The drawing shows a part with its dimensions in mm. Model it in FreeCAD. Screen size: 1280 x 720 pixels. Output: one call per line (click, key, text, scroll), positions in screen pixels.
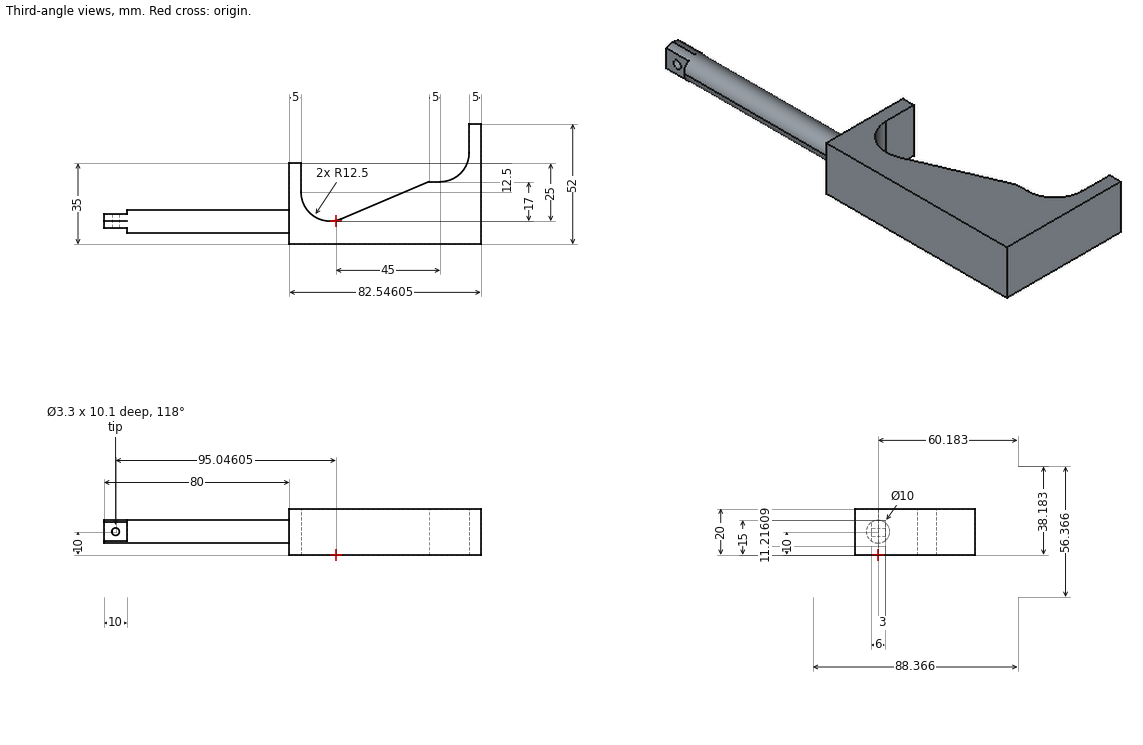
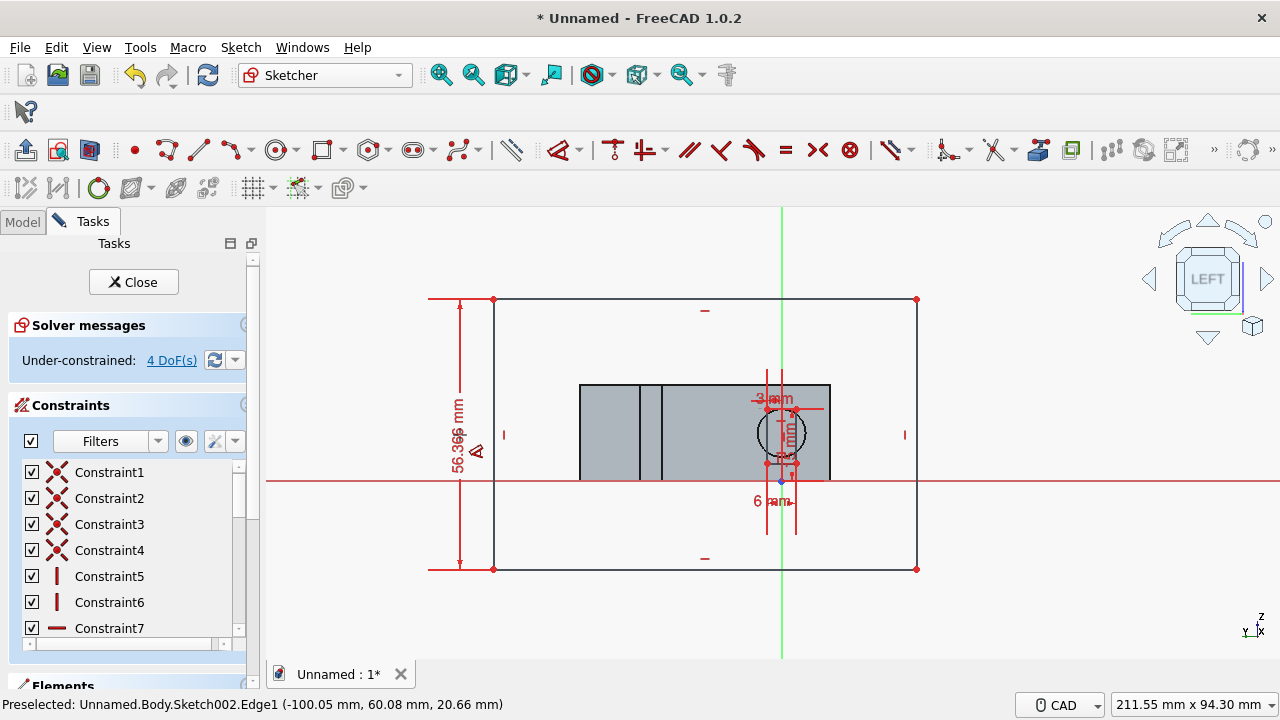
click(621, 570)
click(705, 604)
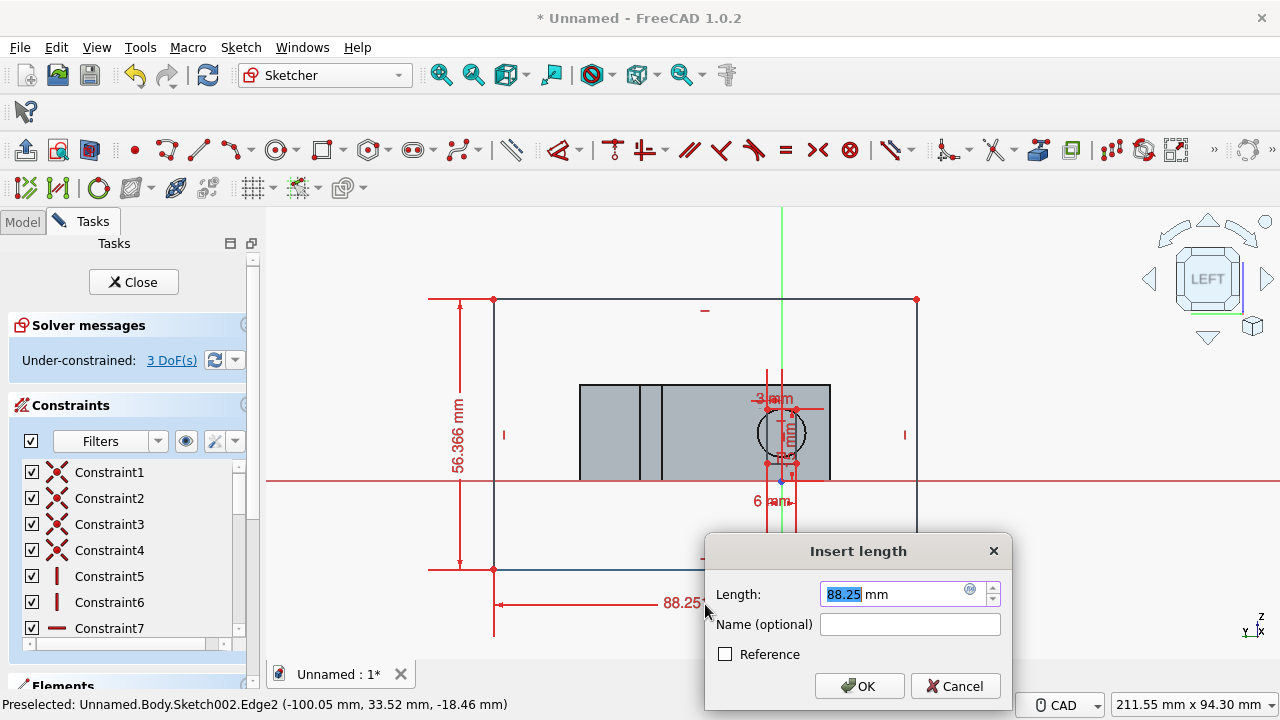
text(88.366)
key(Return)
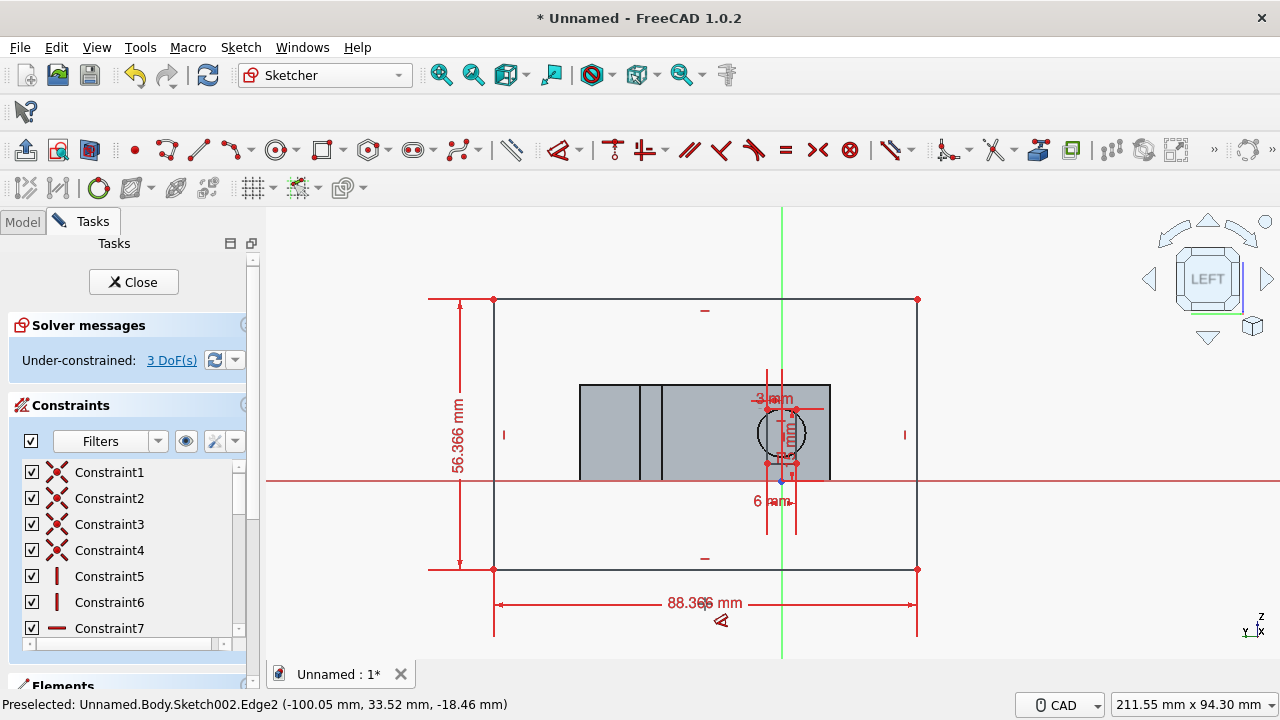
click(494, 299)
click(638, 265)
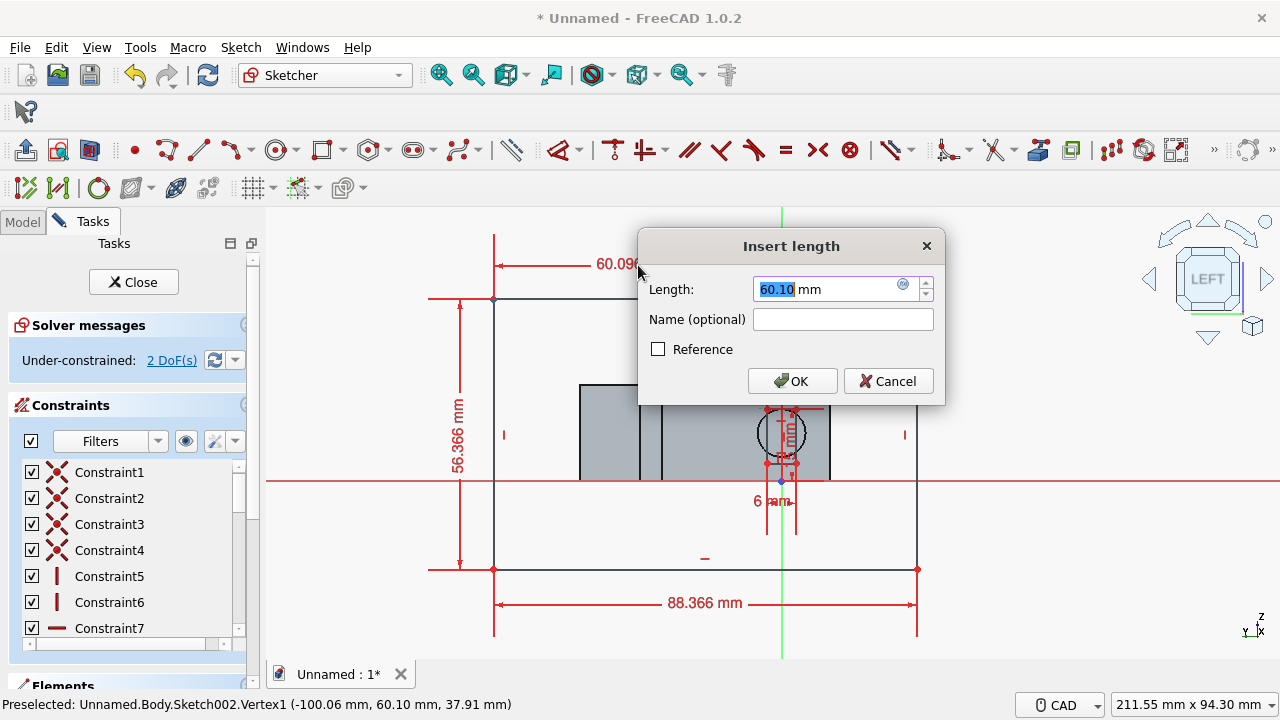
text(60.183)
key(Return)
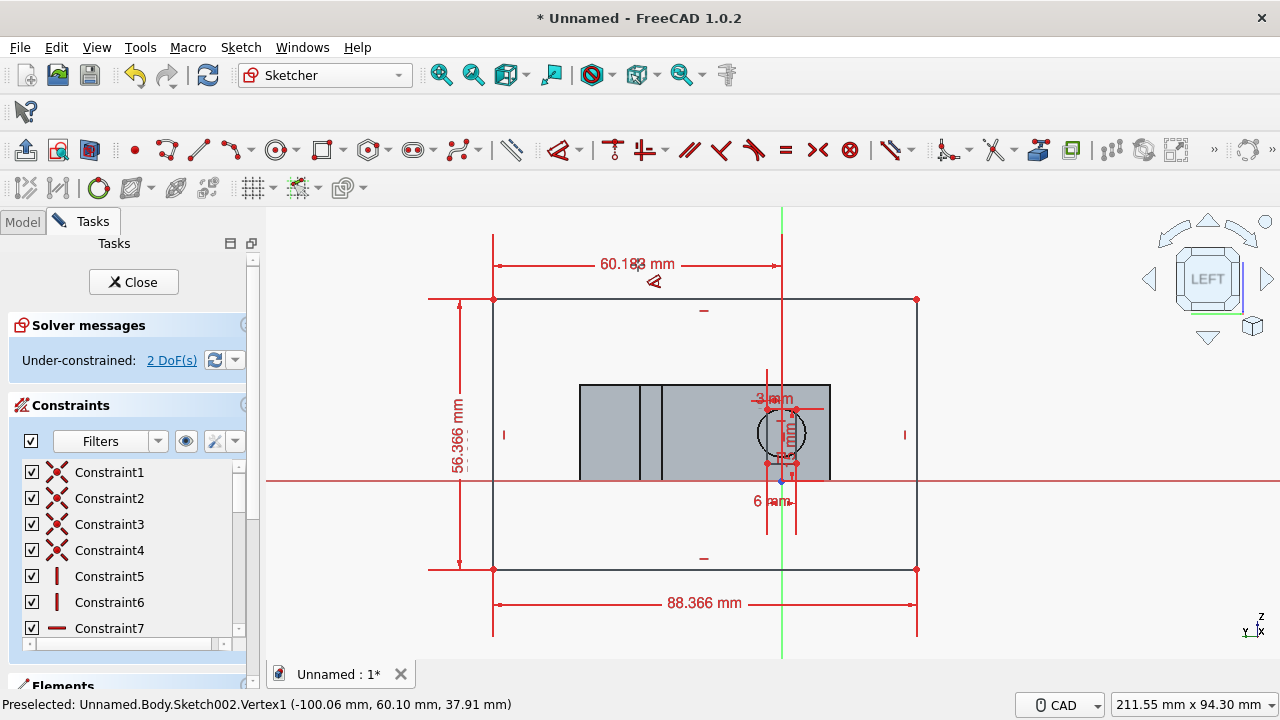
click(493, 299)
click(459, 390)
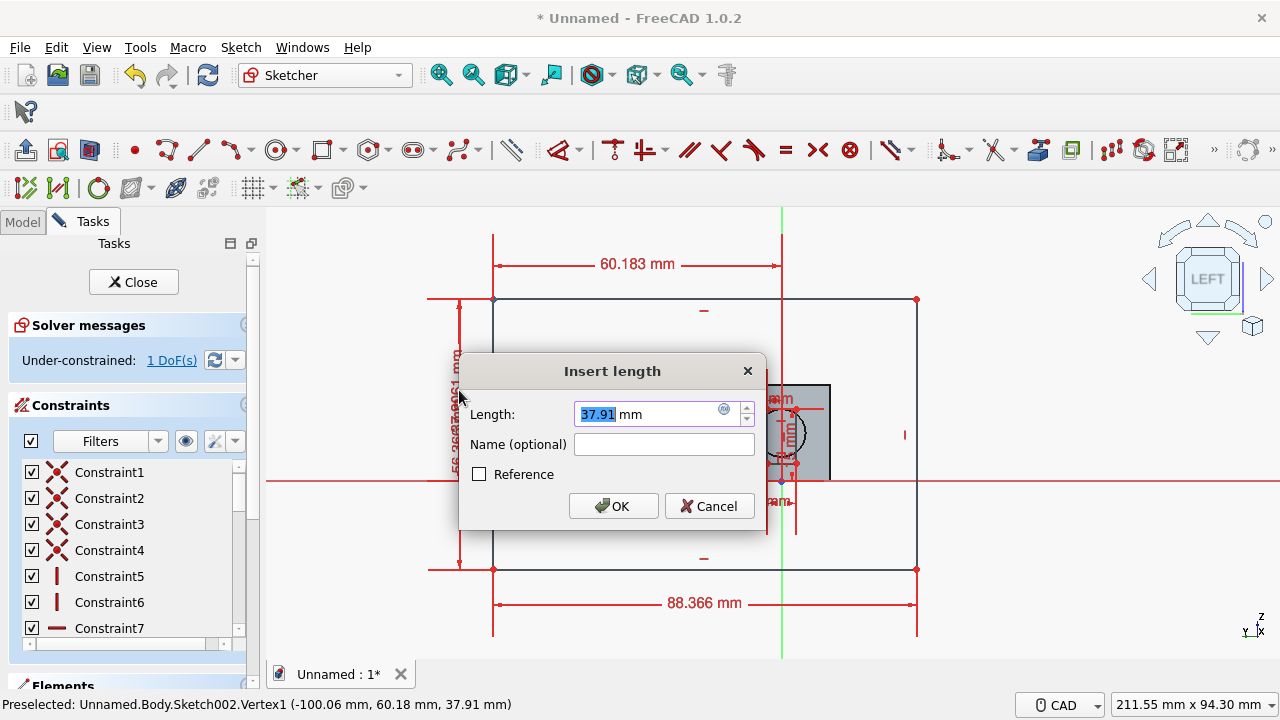
text(38.183)
key(Return)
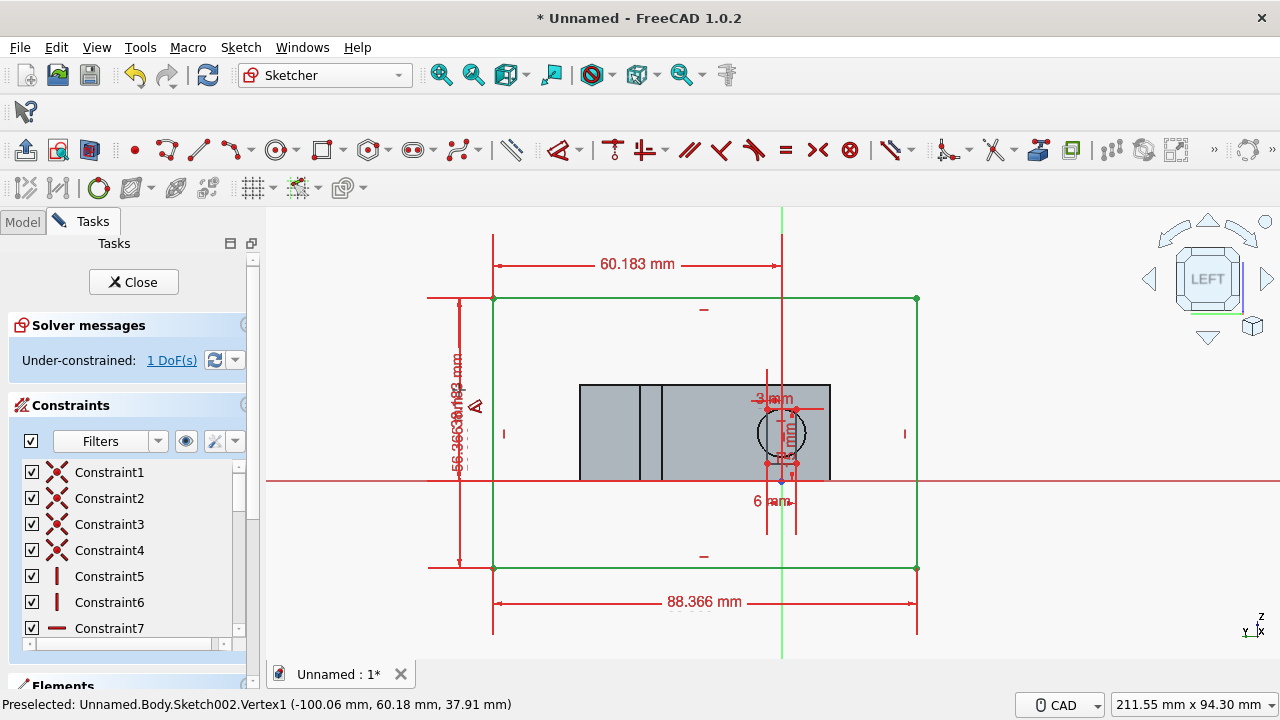
click(767, 425)
click(733, 424)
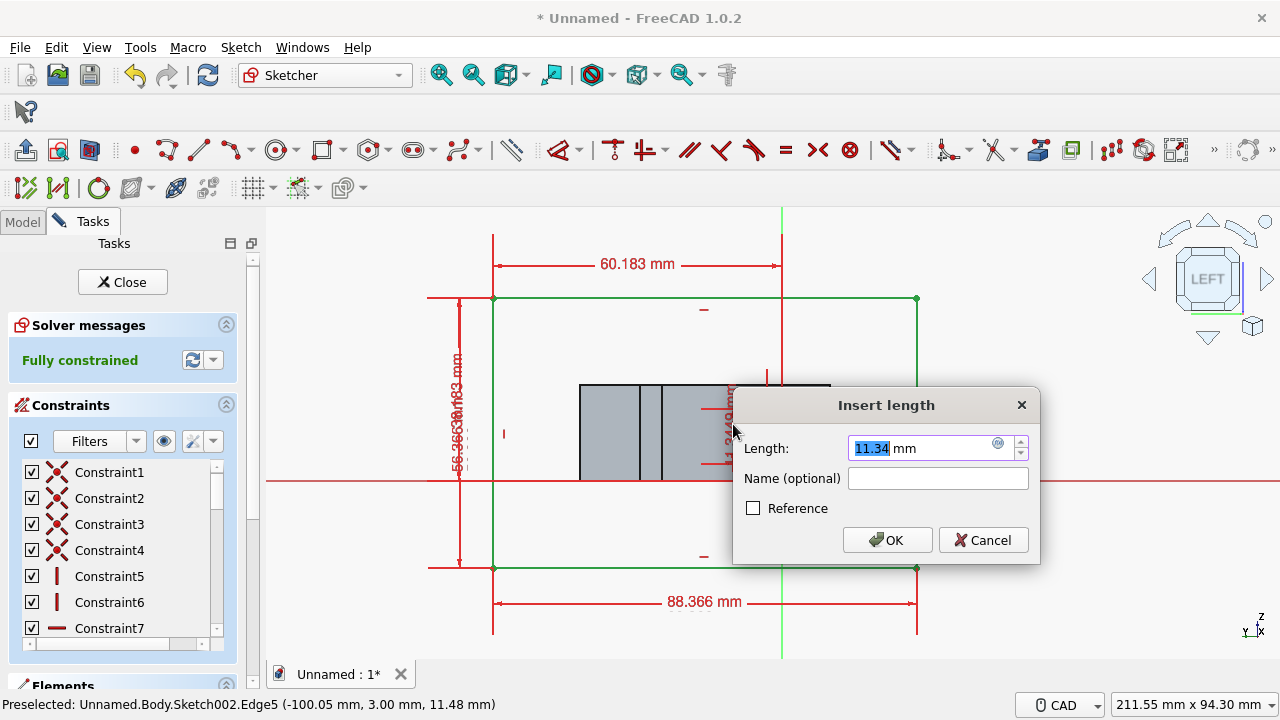
text(11.21609)
key(Return)
key(Escape)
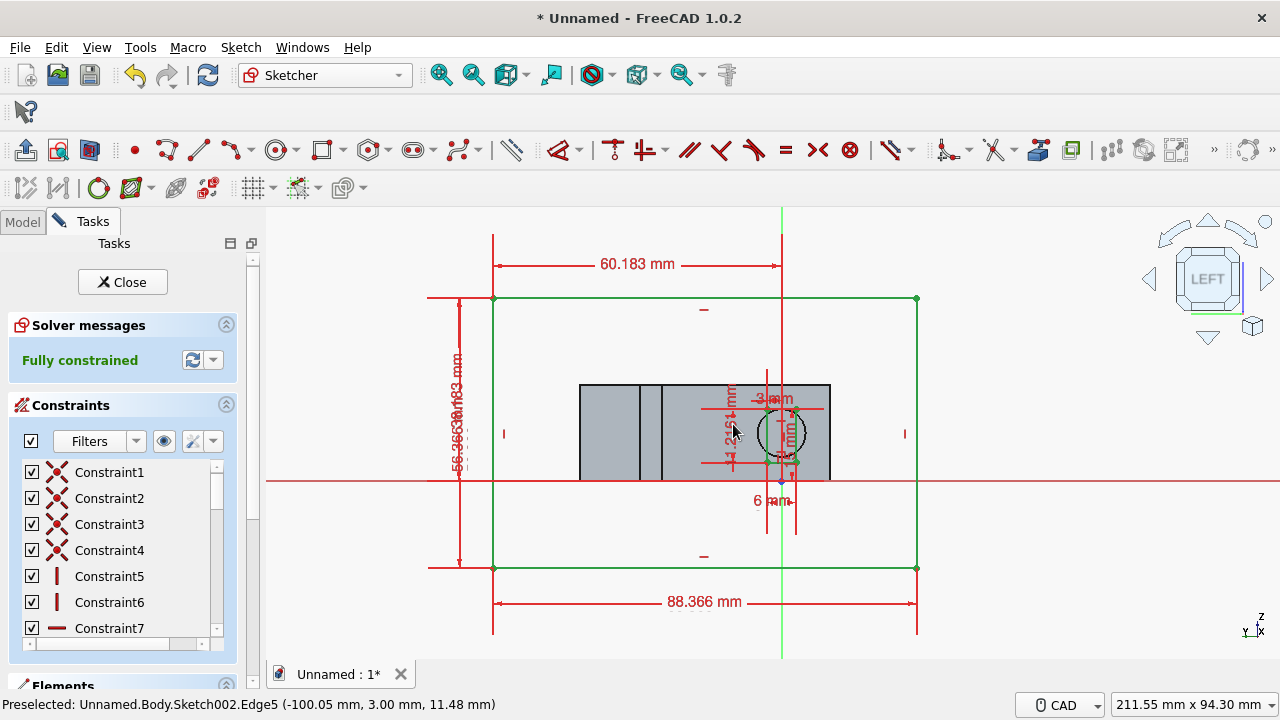
click(123, 282)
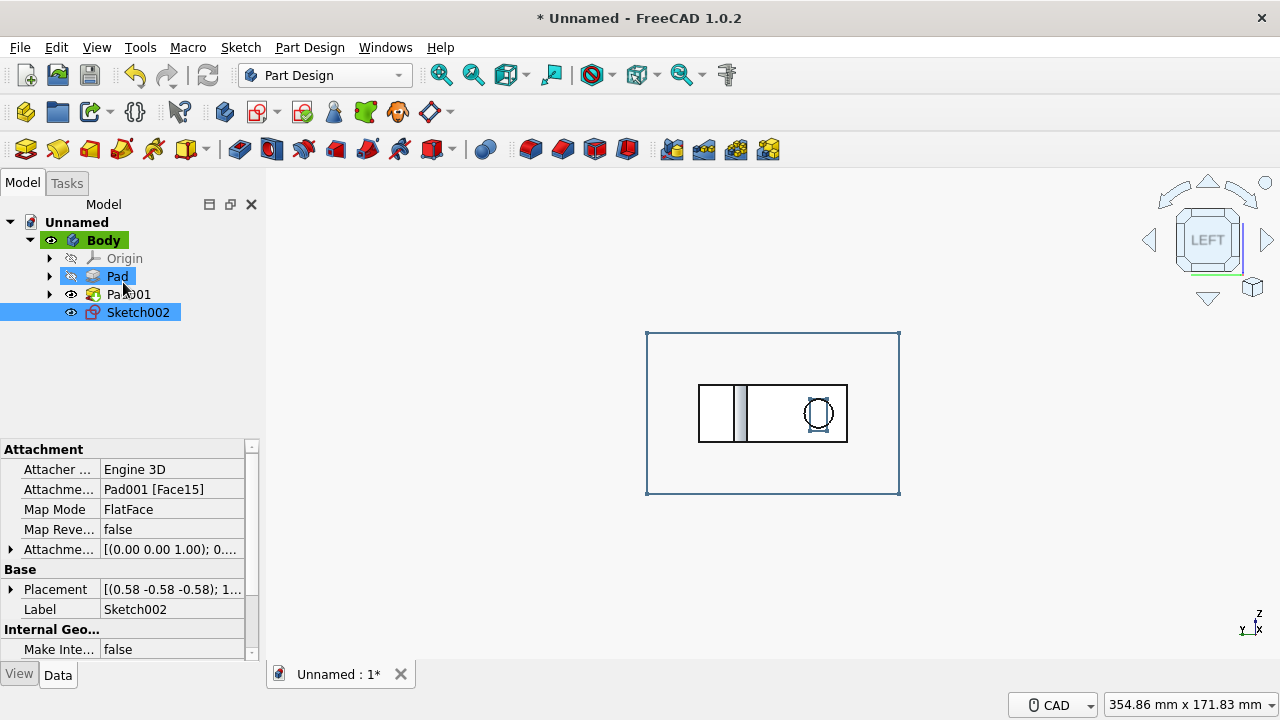
click(240, 150)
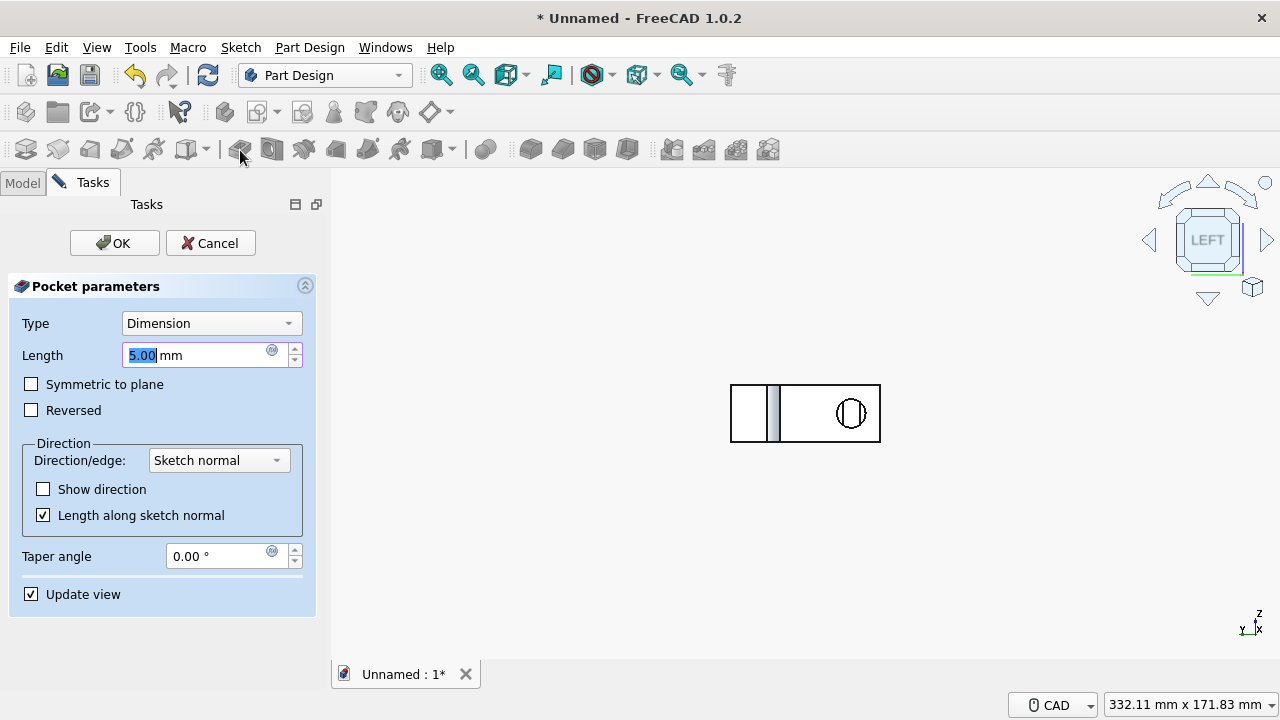
text(10)
key(Tab)